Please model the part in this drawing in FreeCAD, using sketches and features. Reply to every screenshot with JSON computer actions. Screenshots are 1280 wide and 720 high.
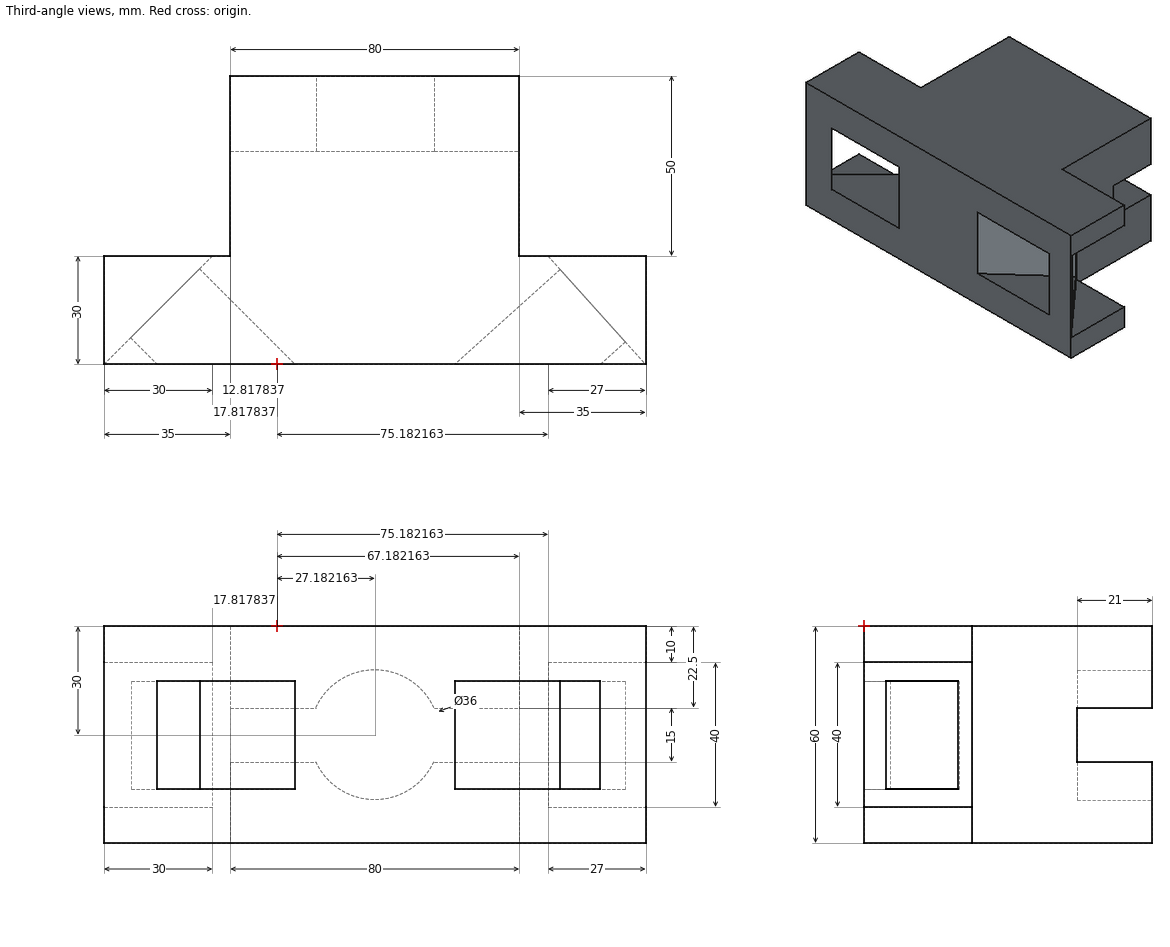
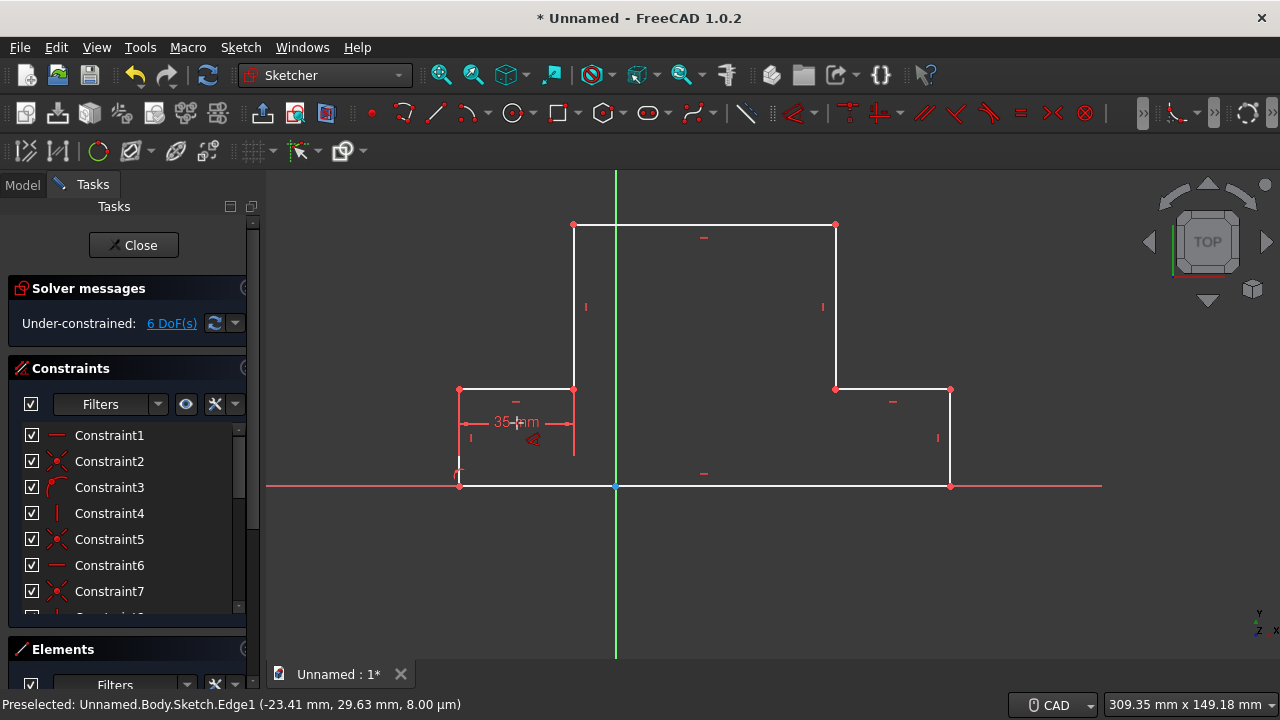
{"action": "left_click", "coordinate": [459, 418]}
{"action": "left_click", "coordinate": [425, 438]}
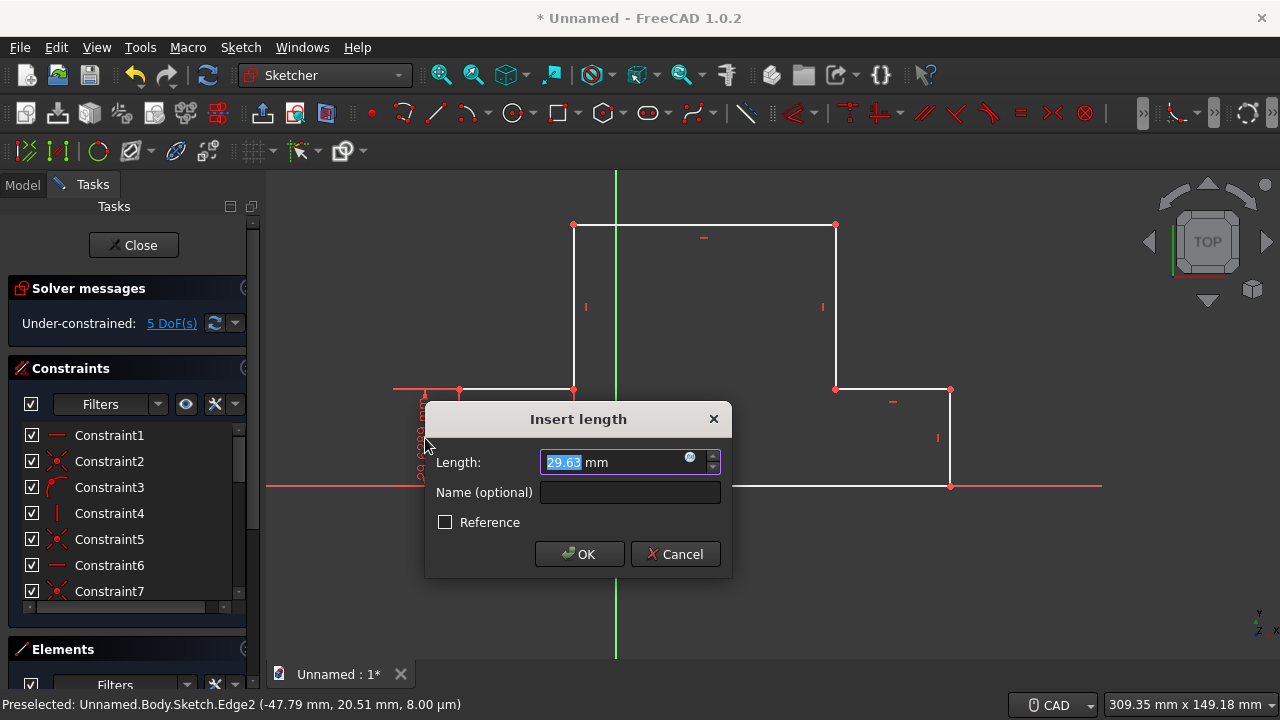
{"action": "type", "text": "30"}
{"action": "key", "text": "Return"}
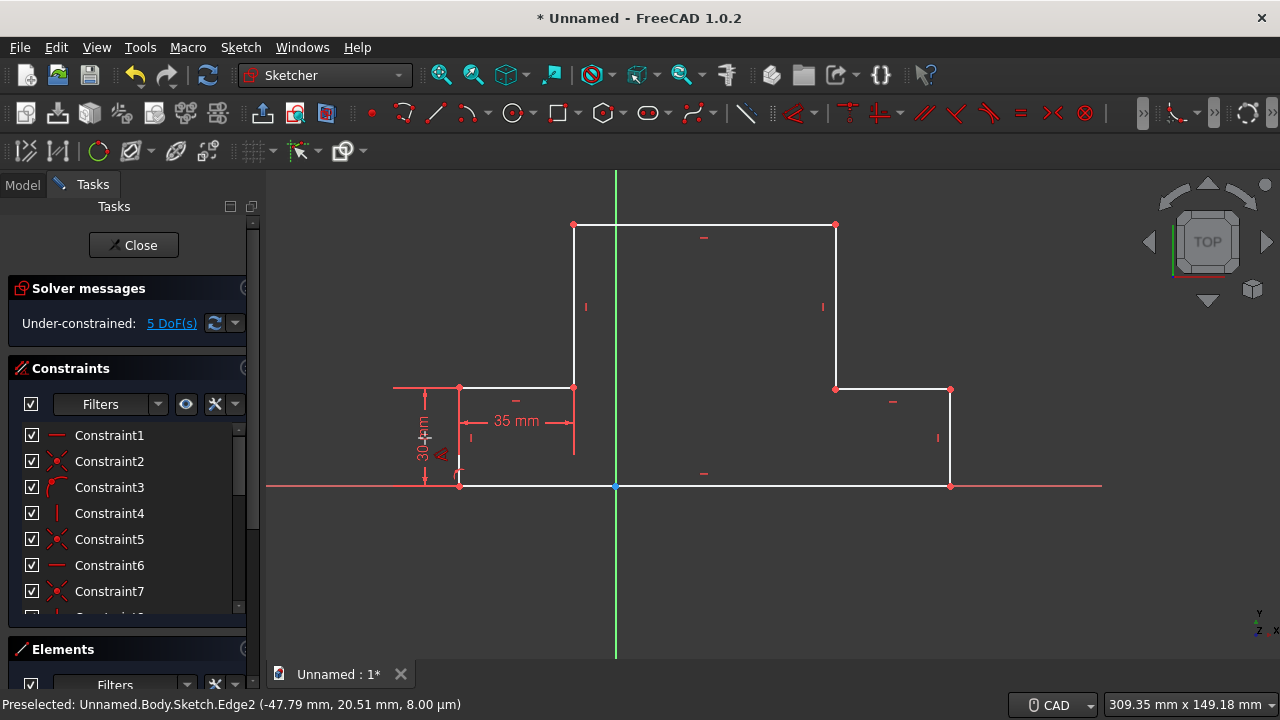
{"action": "left_click", "coordinate": [950, 457]}
{"action": "left_click", "coordinate": [984, 438]}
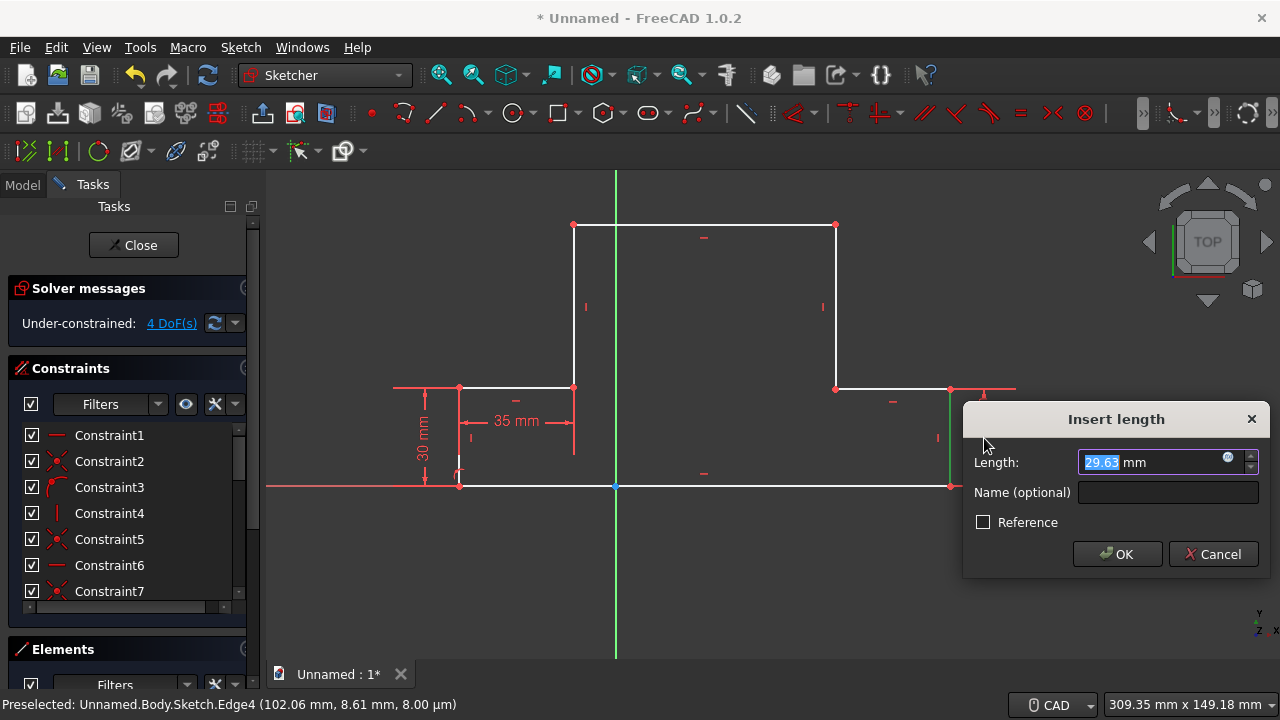
{"action": "type", "text": "30"}
{"action": "key", "text": "Return"}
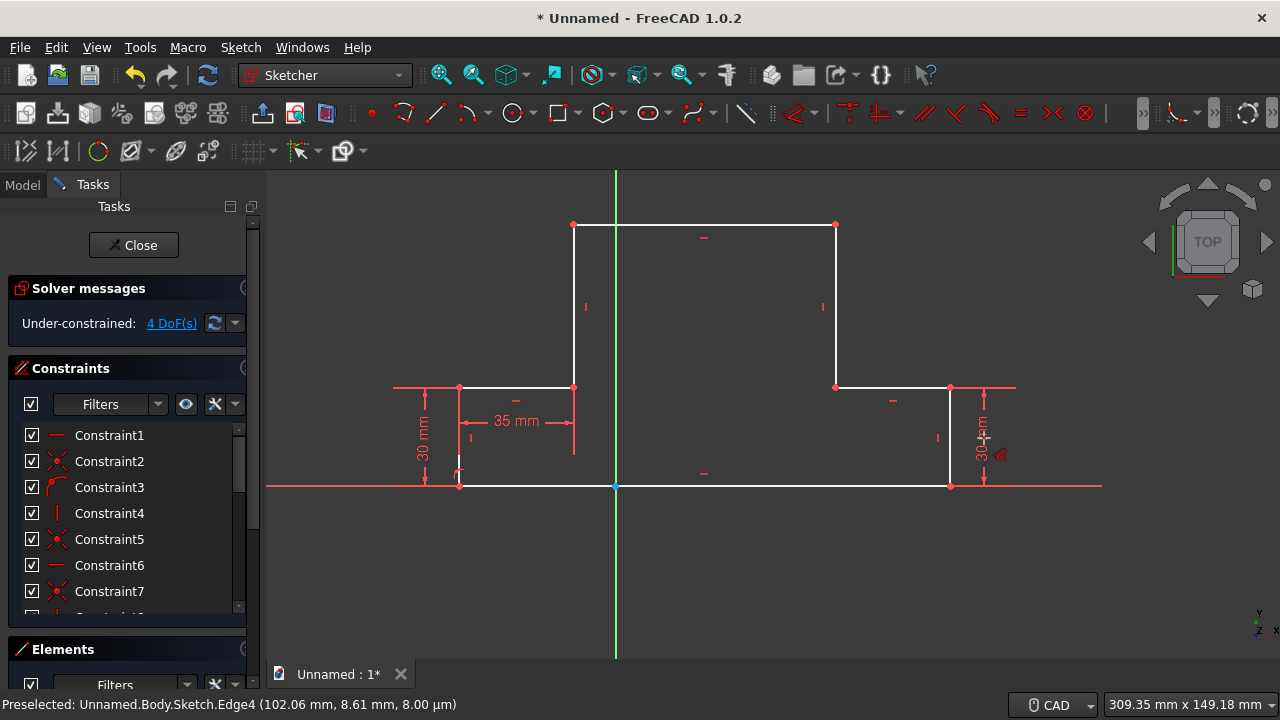
{"action": "left_click", "coordinate": [916, 388]}
{"action": "left_click", "coordinate": [893, 422]}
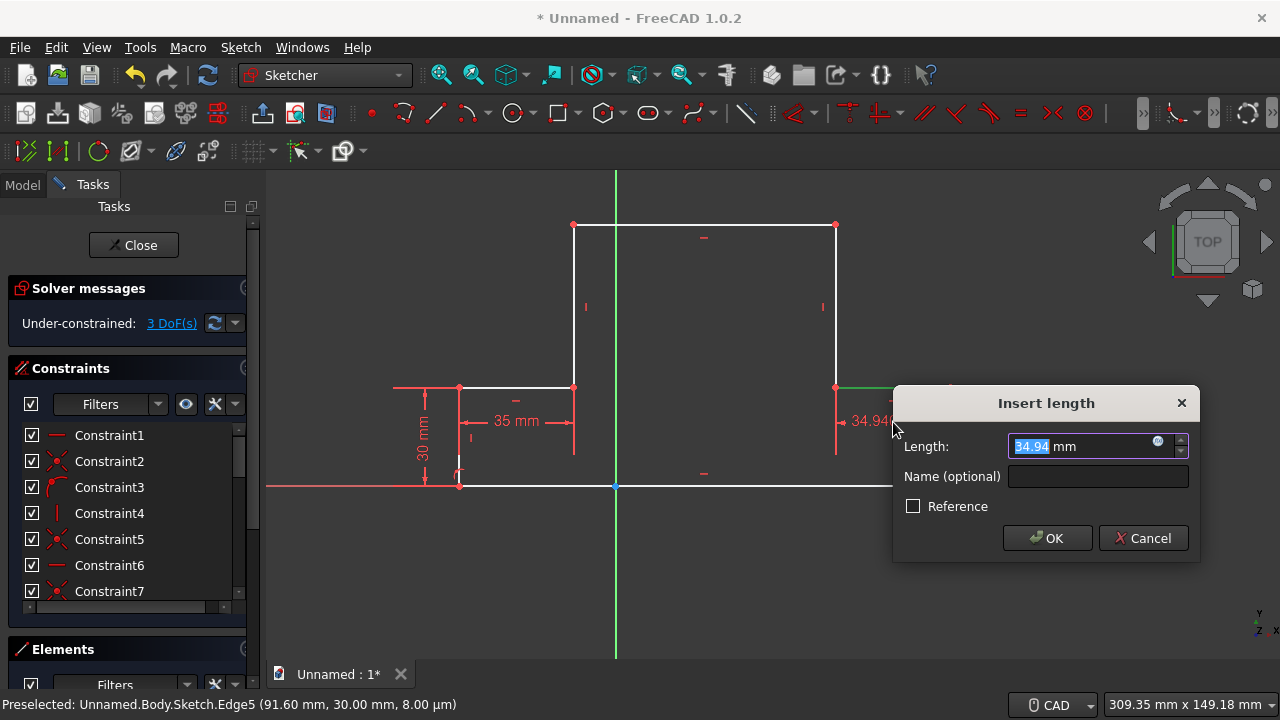
{"action": "type", "text": "35"}
{"action": "key", "text": "Return"}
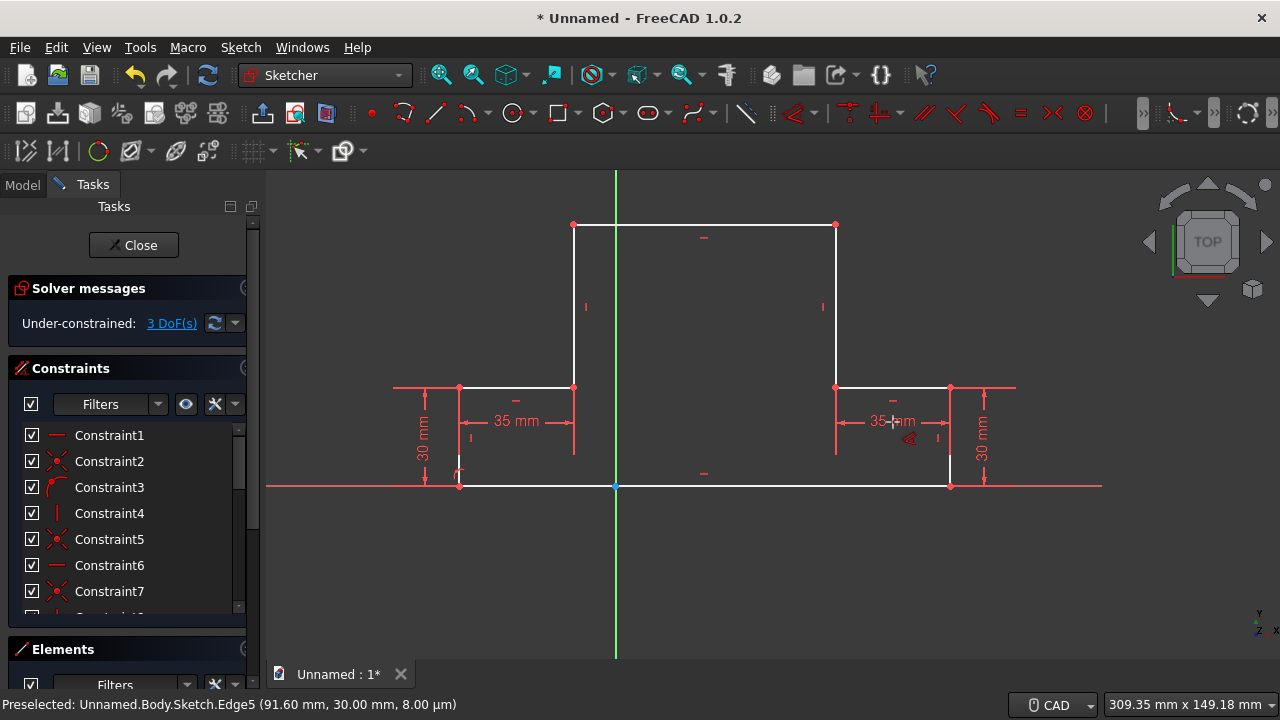
{"action": "left_click", "coordinate": [836, 339]}
{"action": "left_click", "coordinate": [870, 306]}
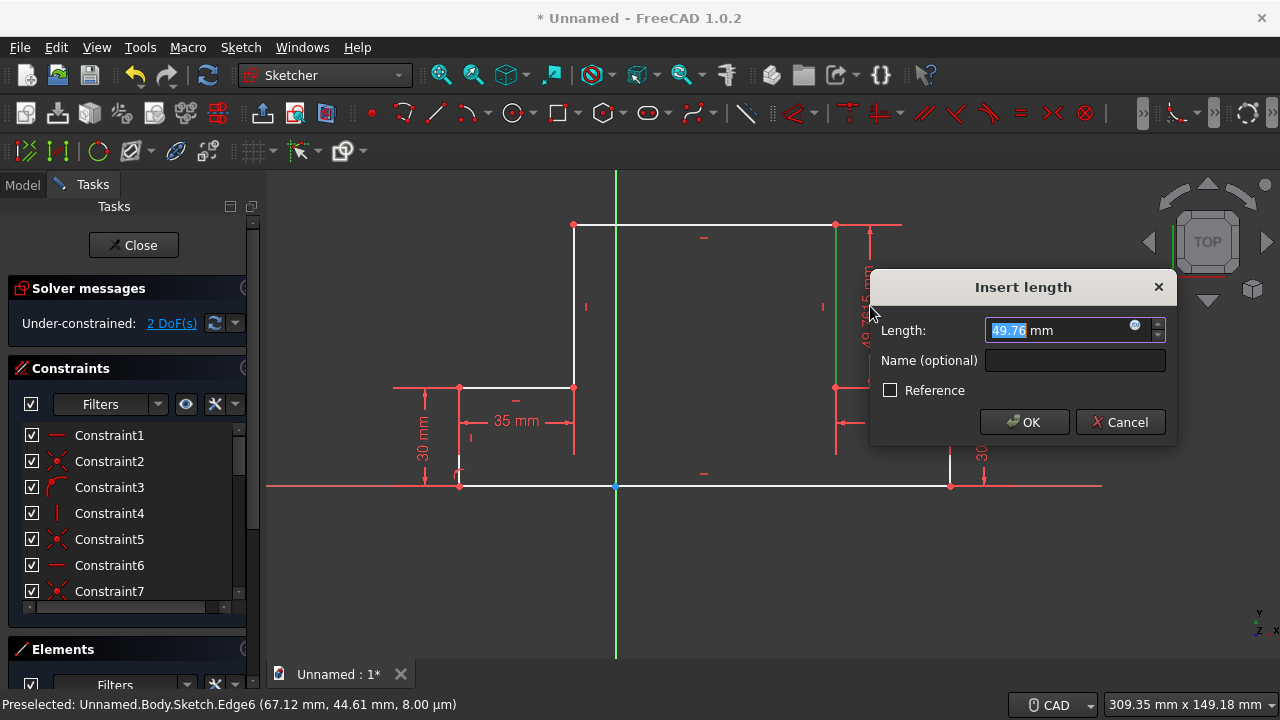
{"action": "type", "text": "50"}
{"action": "key", "text": "Return"}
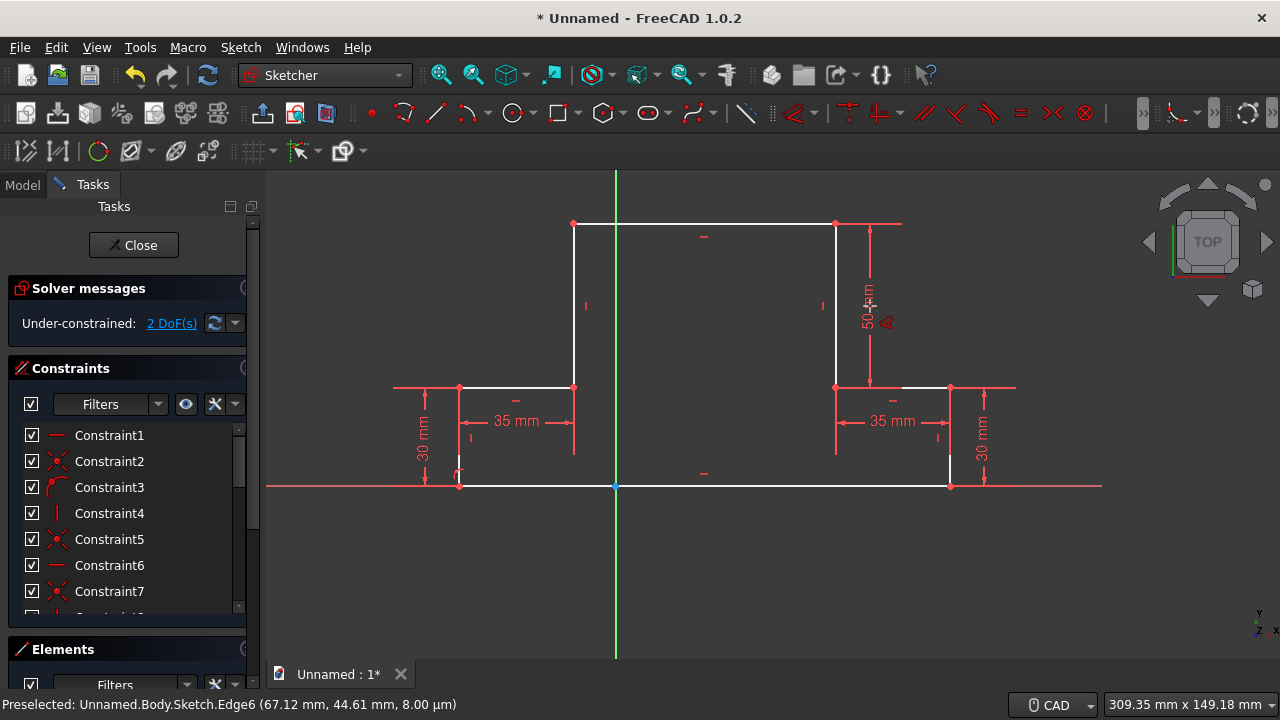
{"action": "left_click", "coordinate": [757, 224]}
{"action": "left_click", "coordinate": [705, 258]}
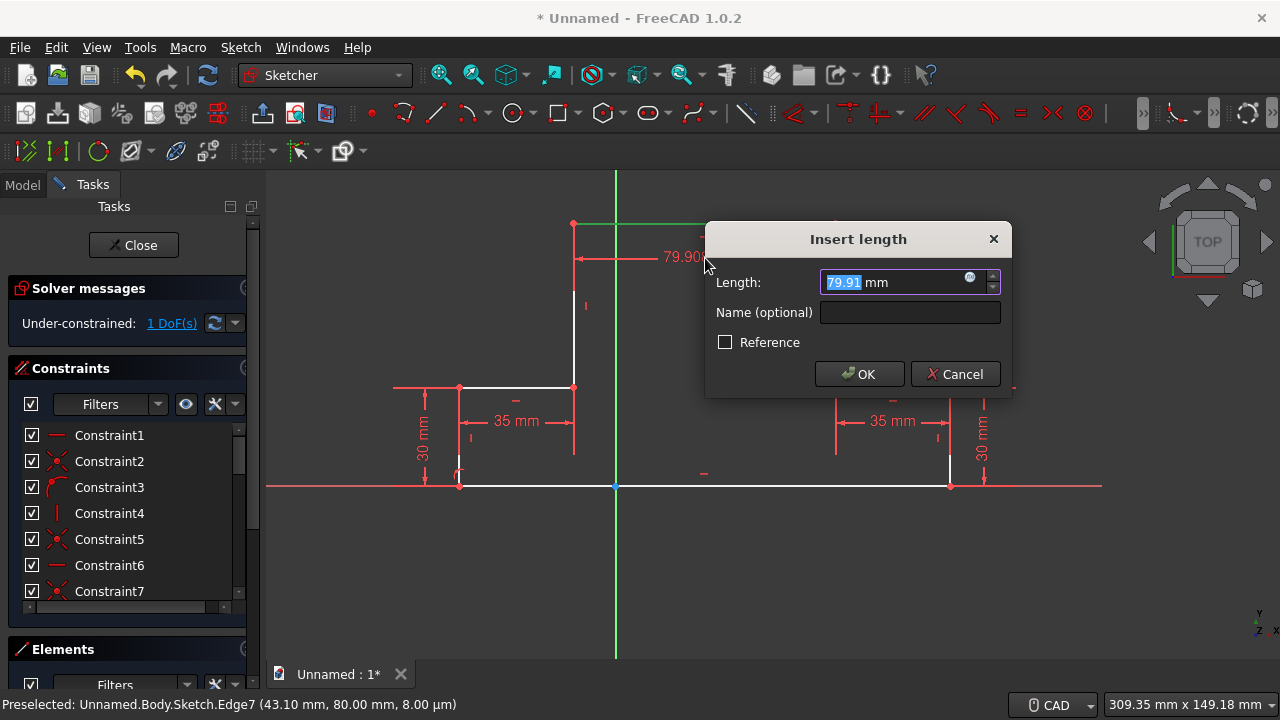
{"action": "type", "text": "80"}
{"action": "key", "text": "Return"}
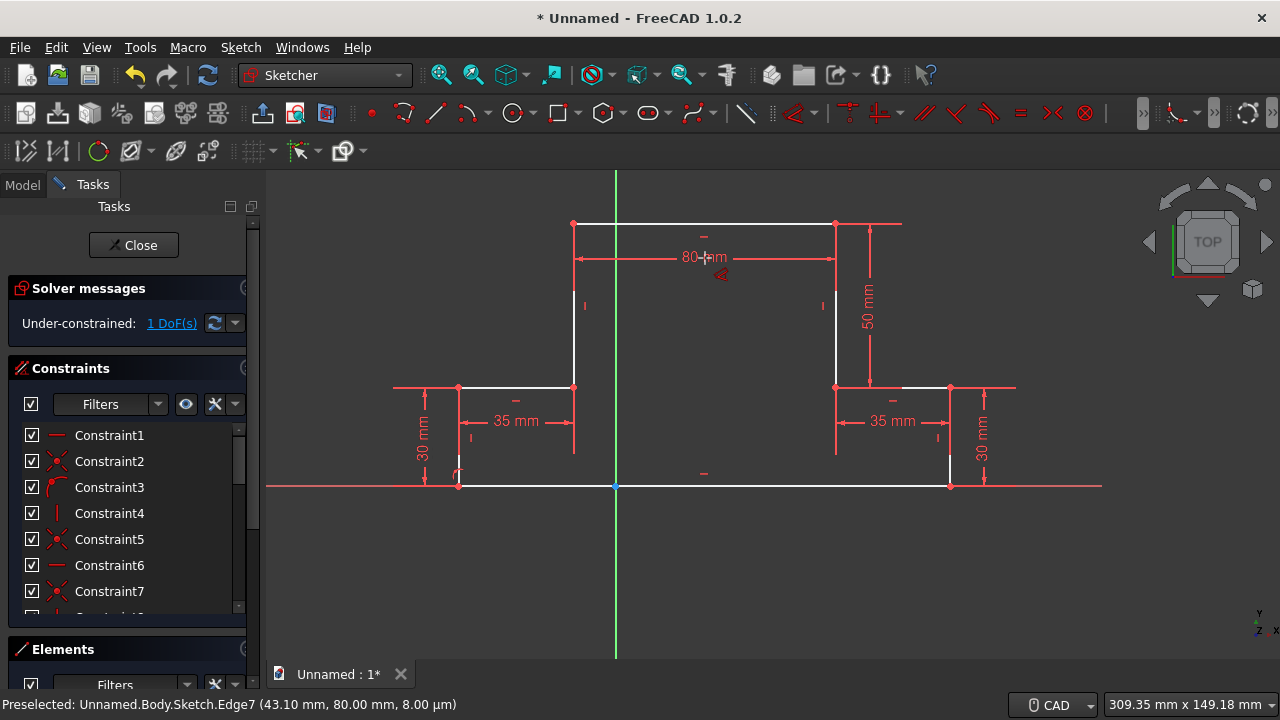
{"action": "left_click", "coordinate": [574, 388]}
{"action": "left_click", "coordinate": [595, 520]}